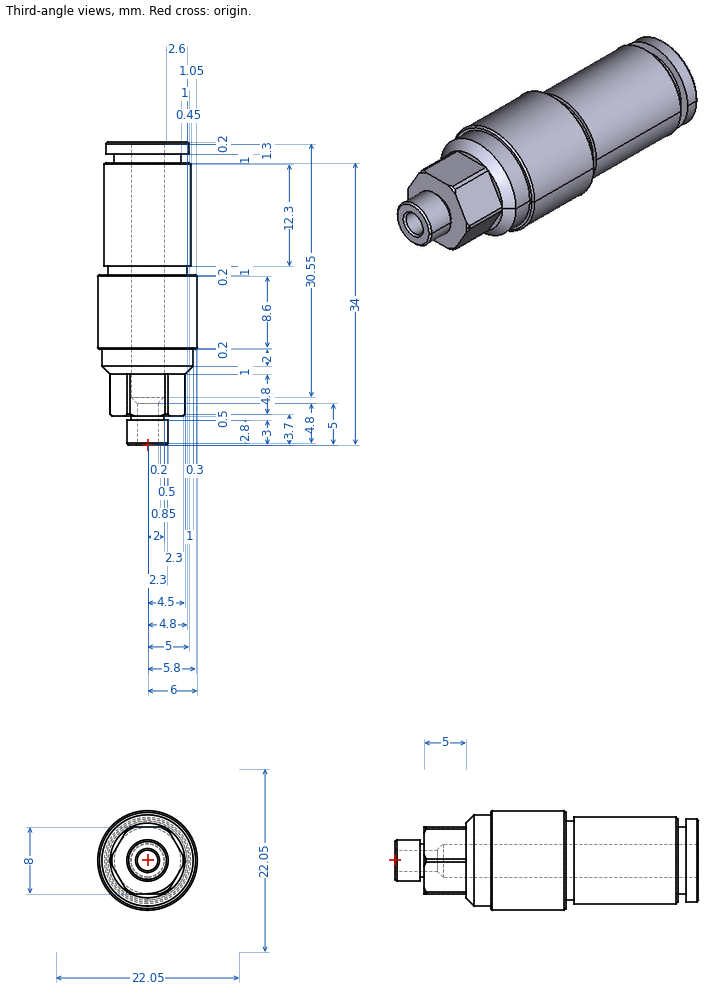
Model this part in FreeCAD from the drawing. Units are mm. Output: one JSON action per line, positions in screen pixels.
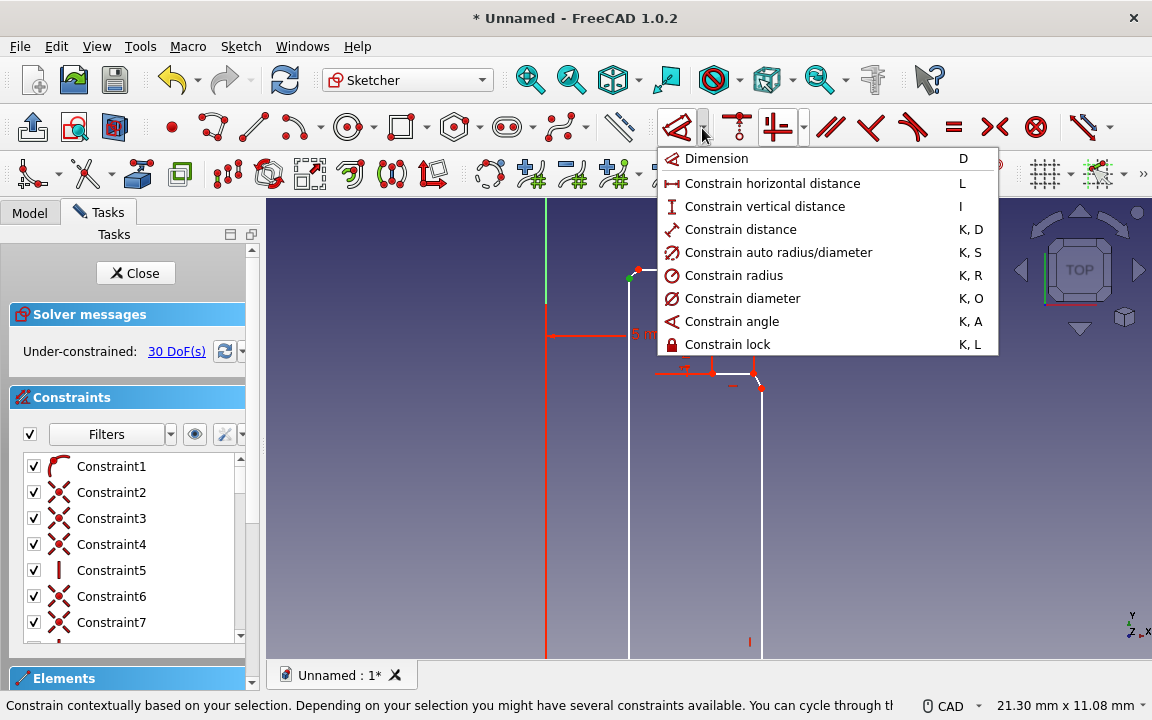
{"action": "left_click", "coordinate": [828, 184]}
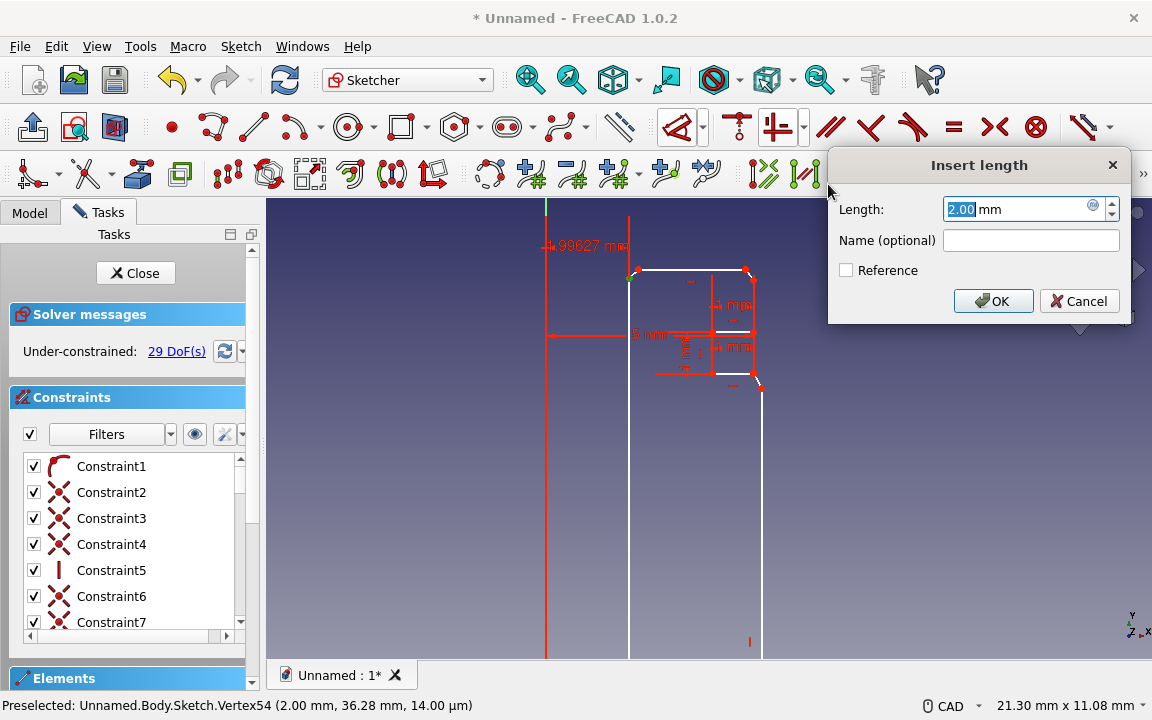
{"action": "type", "text": "2"}
{"action": "key", "text": "Return"}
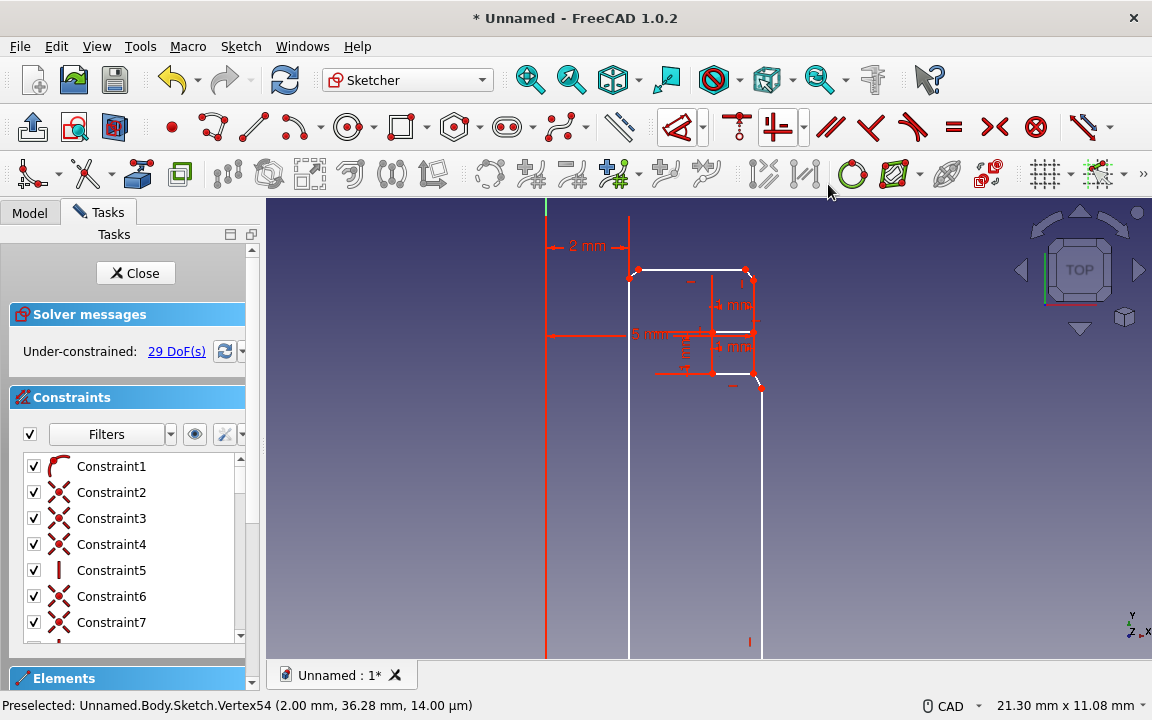
{"action": "scroll", "coordinate": [633, 277], "scroll_direction": "down", "scroll_amount": 8}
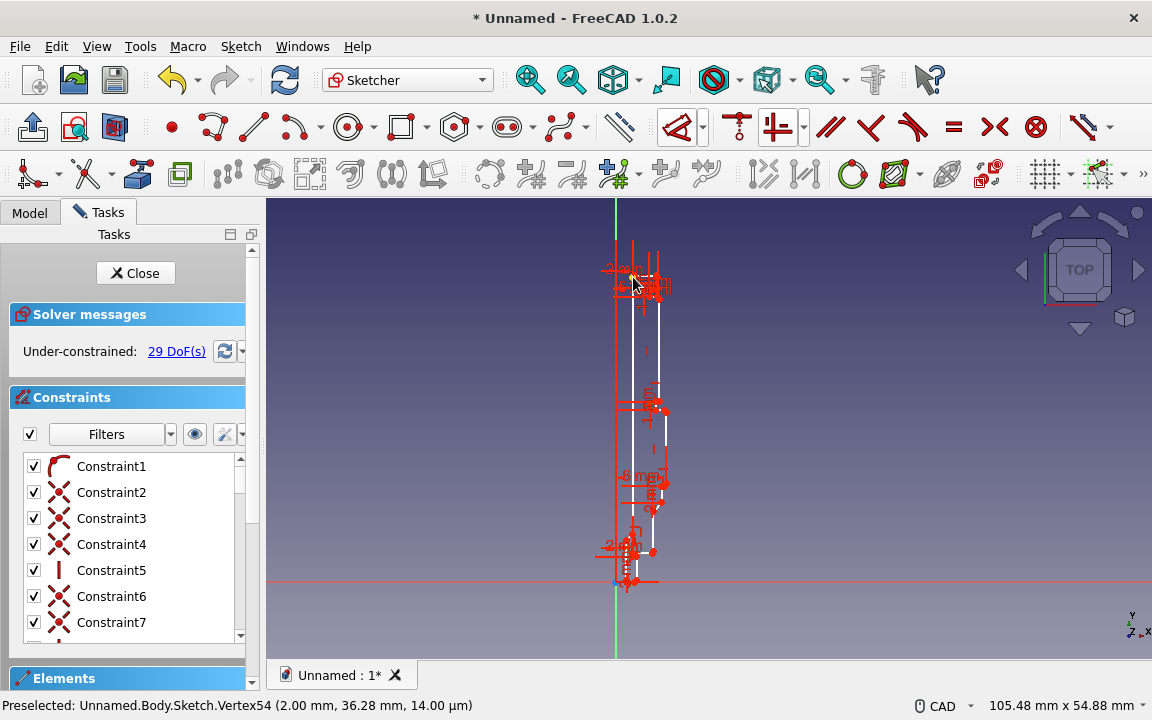
{"action": "scroll", "coordinate": [626, 541], "scroll_direction": "up", "scroll_amount": 2}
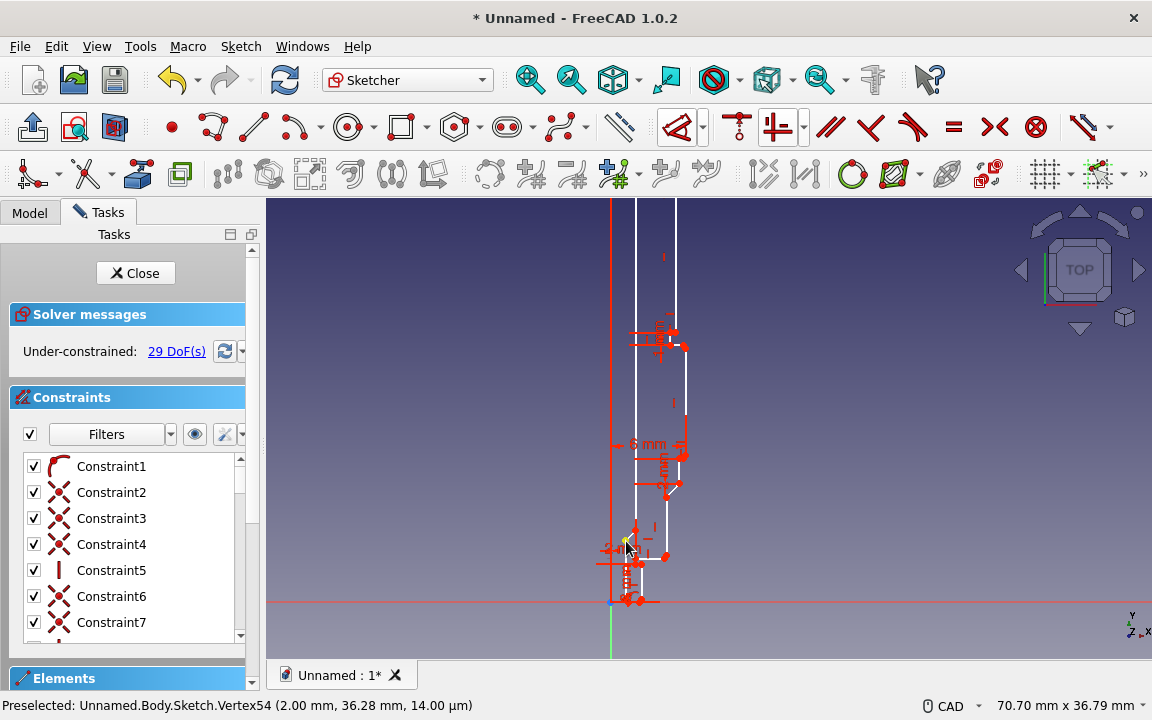
{"action": "left_click", "coordinate": [626, 540]}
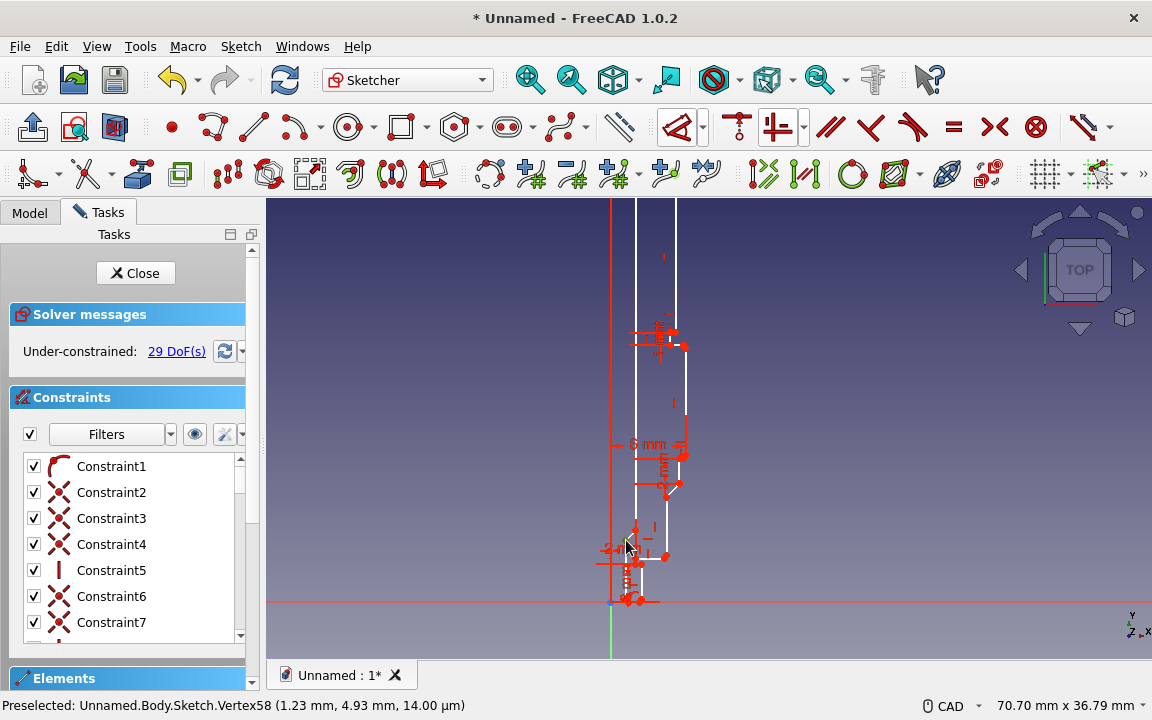
{"action": "left_click", "coordinate": [702, 128]}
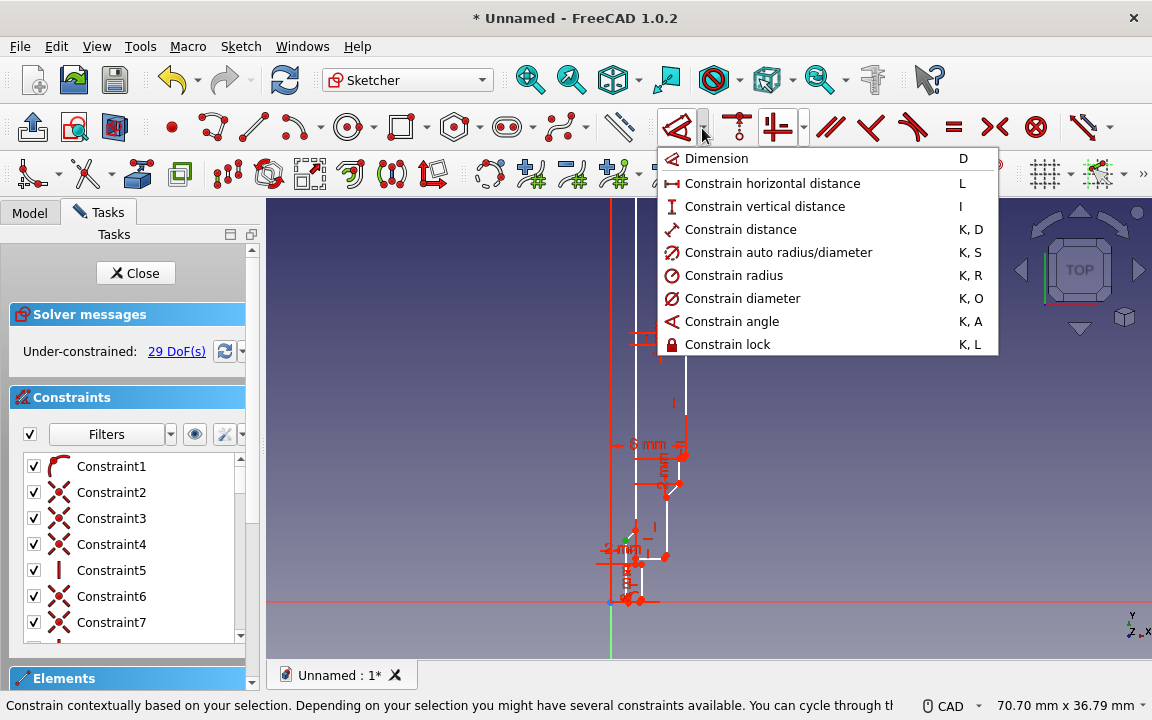
{"action": "left_click", "coordinate": [828, 206]}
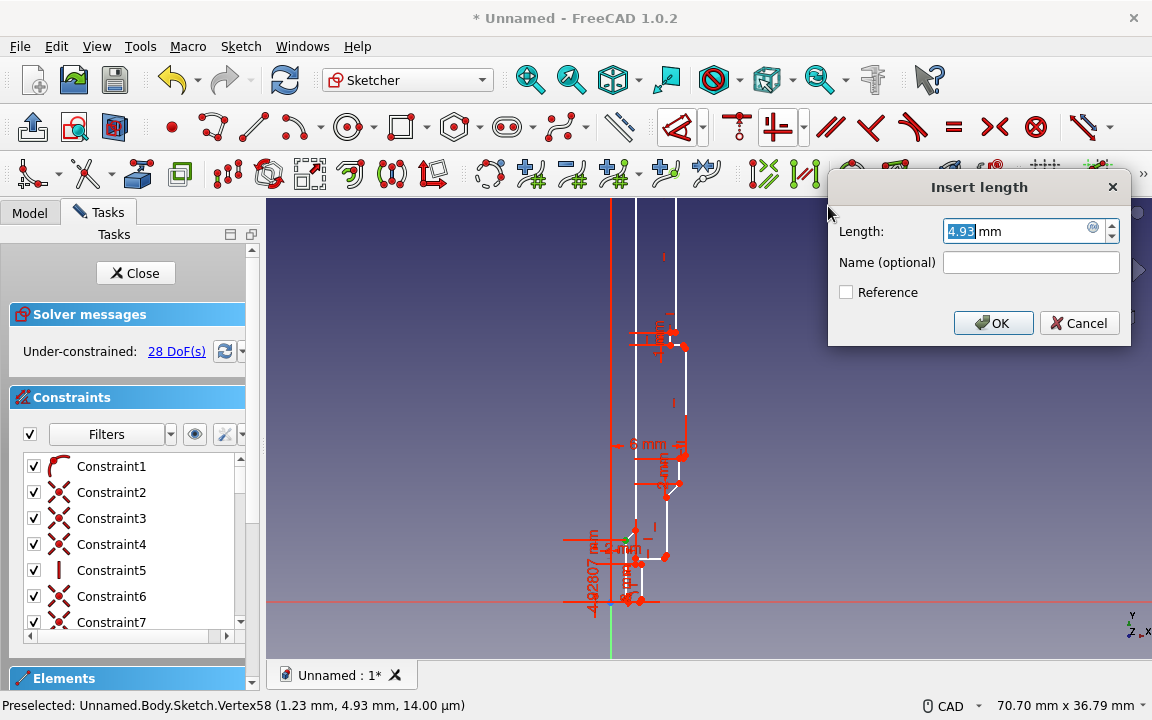
{"action": "type", "text": "5"}
{"action": "key", "text": "Return"}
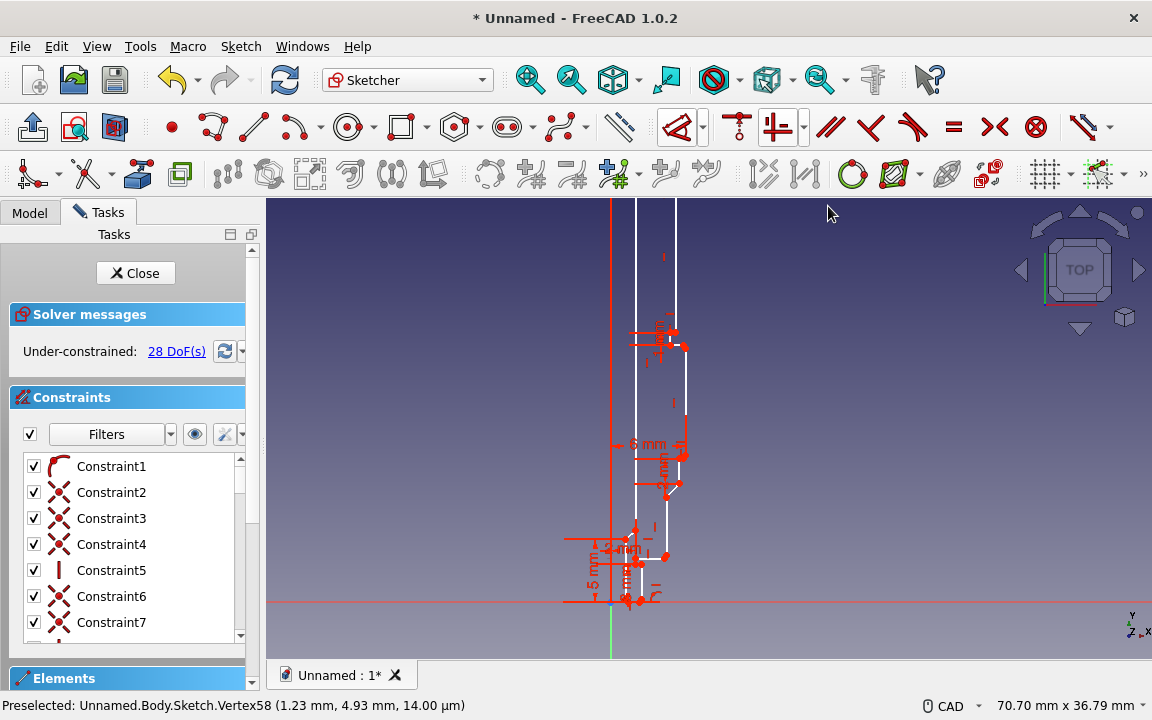
{"action": "scroll", "coordinate": [673, 490], "scroll_direction": "up", "scroll_amount": 6}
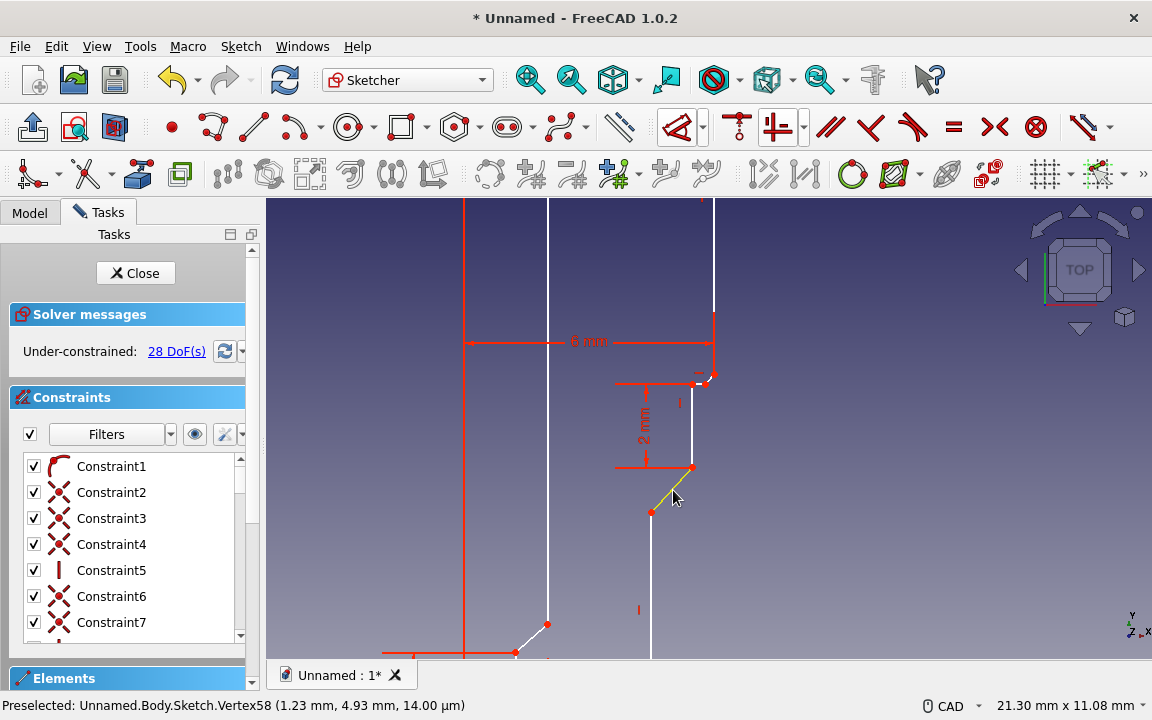
{"action": "left_click", "coordinate": [672, 490]}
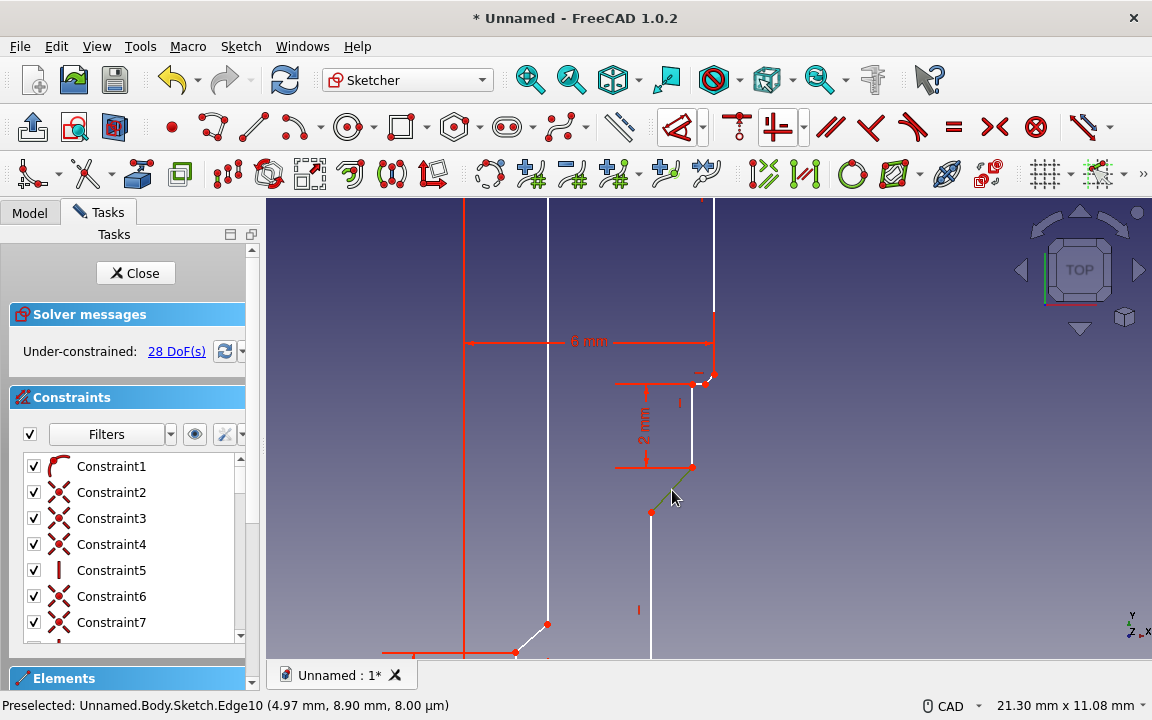
{"action": "key", "text": "l"}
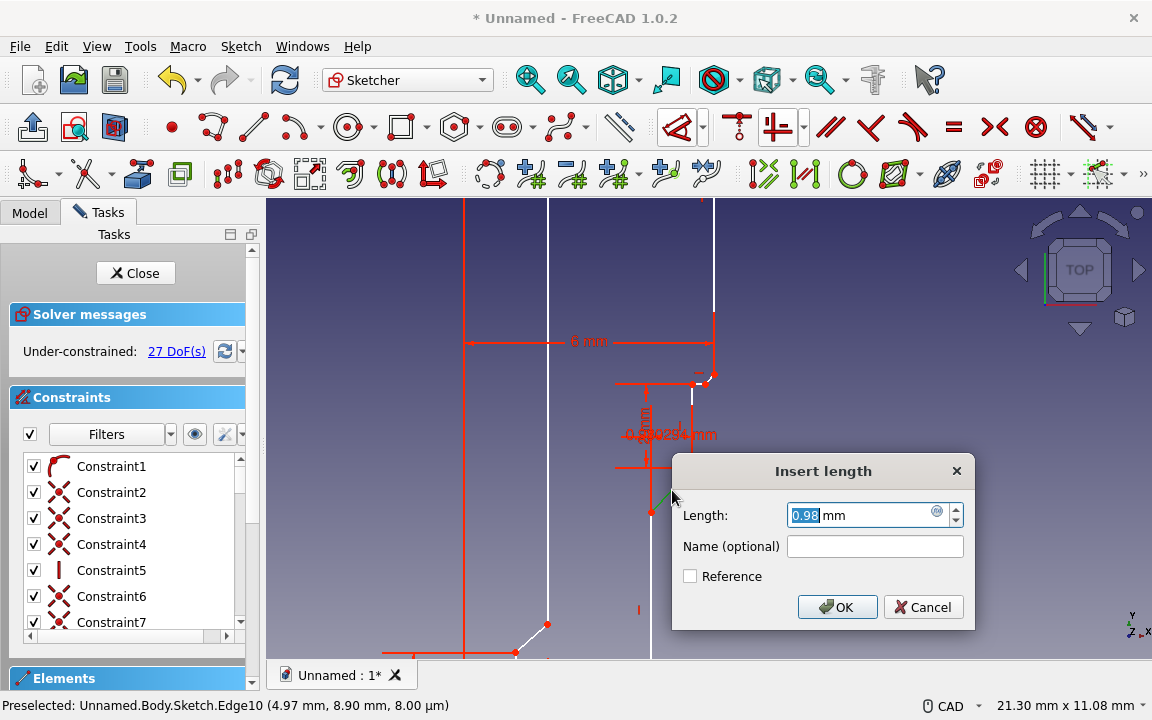
{"action": "type", "text": "1"}
{"action": "key", "text": "Return"}